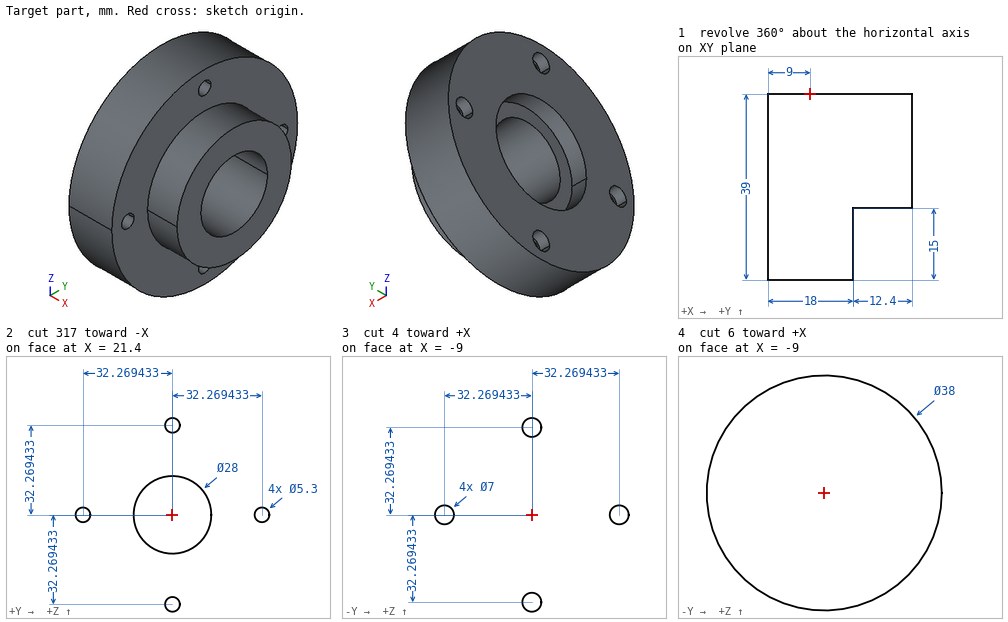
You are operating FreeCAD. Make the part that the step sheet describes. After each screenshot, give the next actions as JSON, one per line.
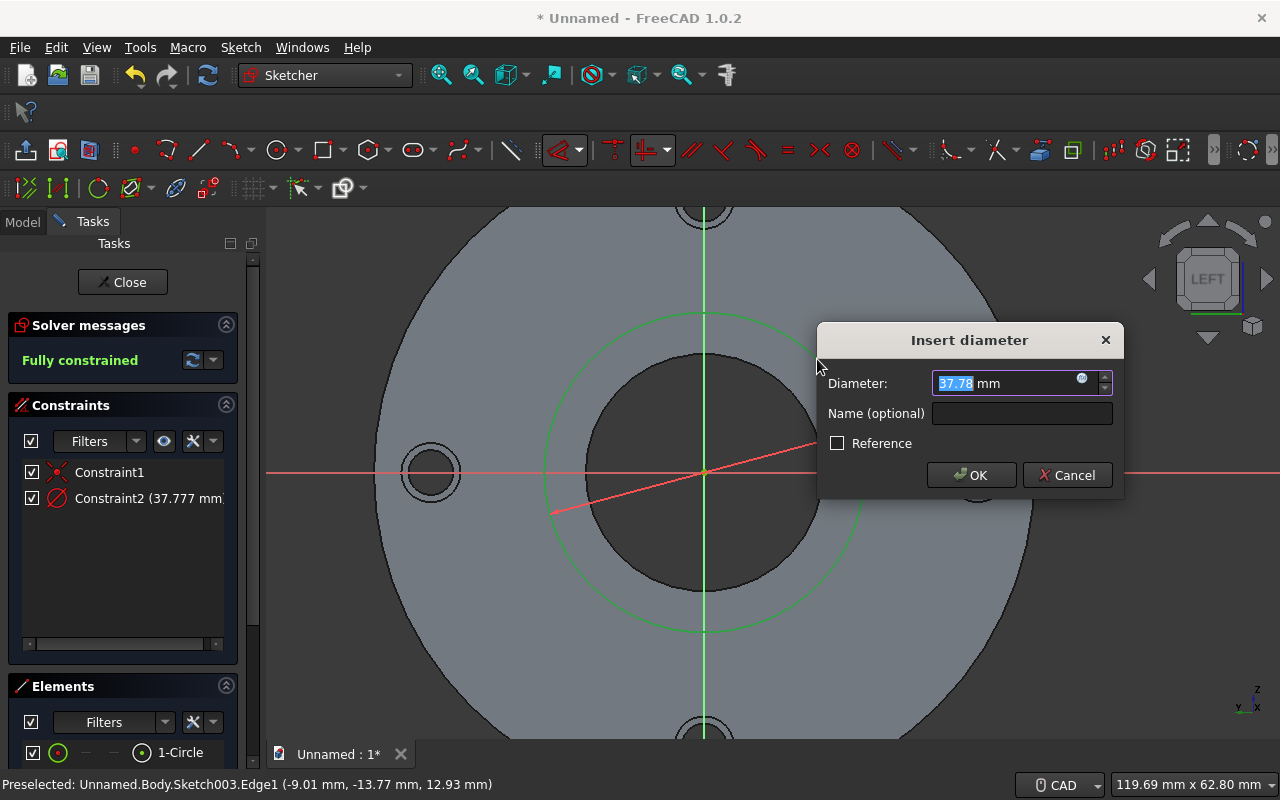
{"action": "type", "text": "38"}
{"action": "key", "text": "Return"}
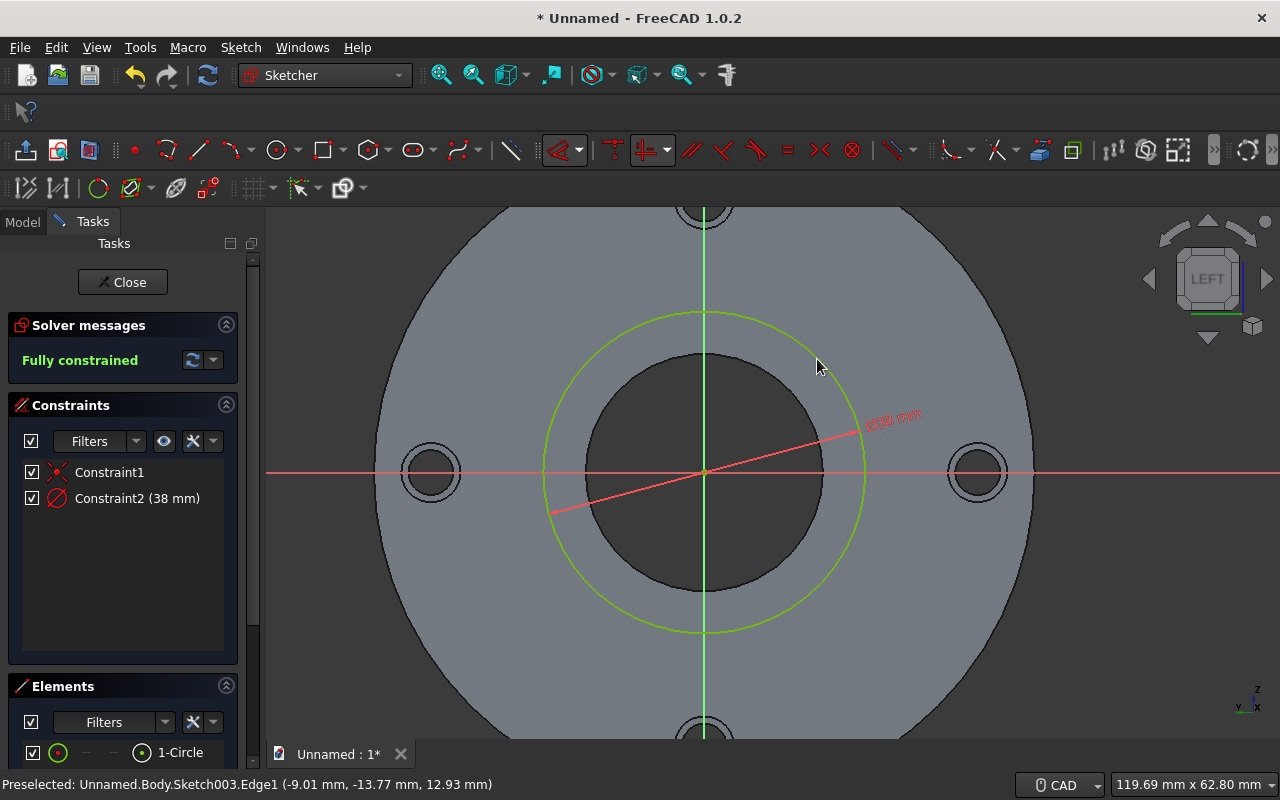
{"action": "left_click", "coordinate": [123, 282]}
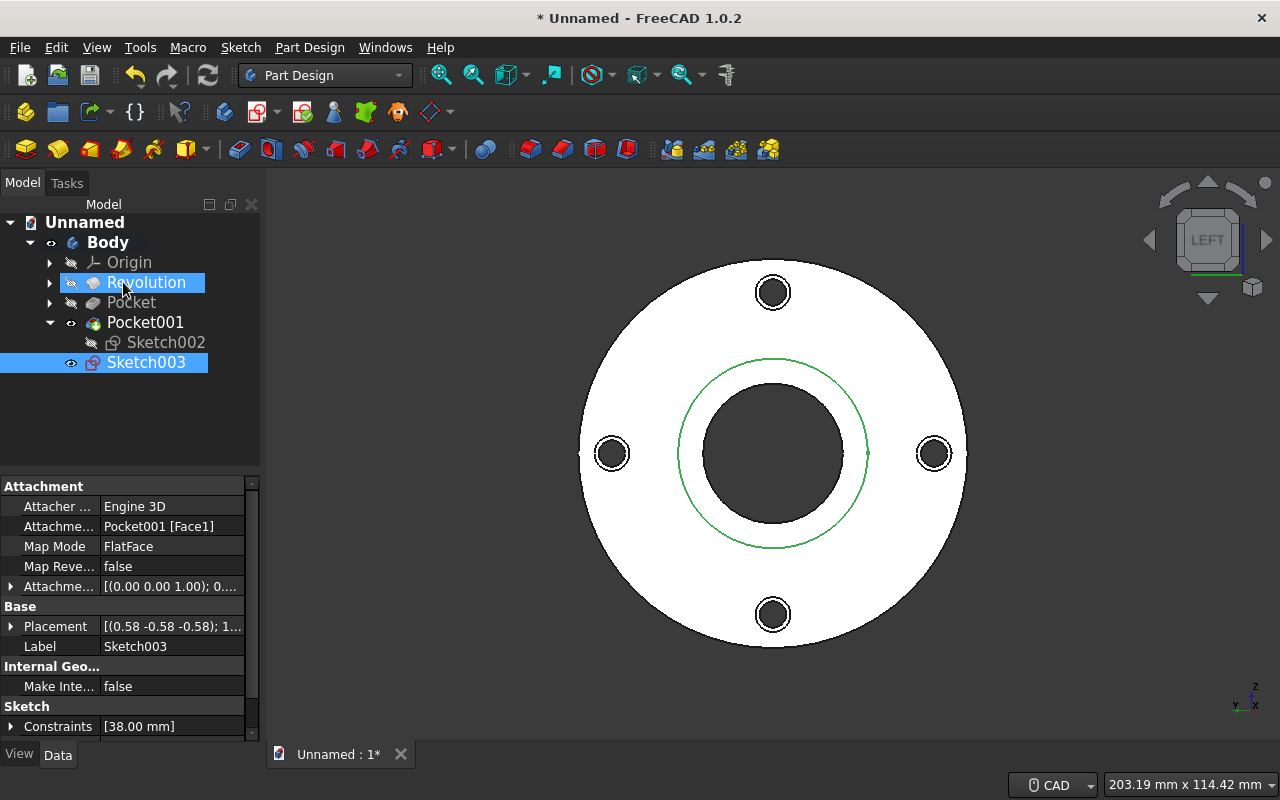
{"action": "left_click", "coordinate": [240, 150]}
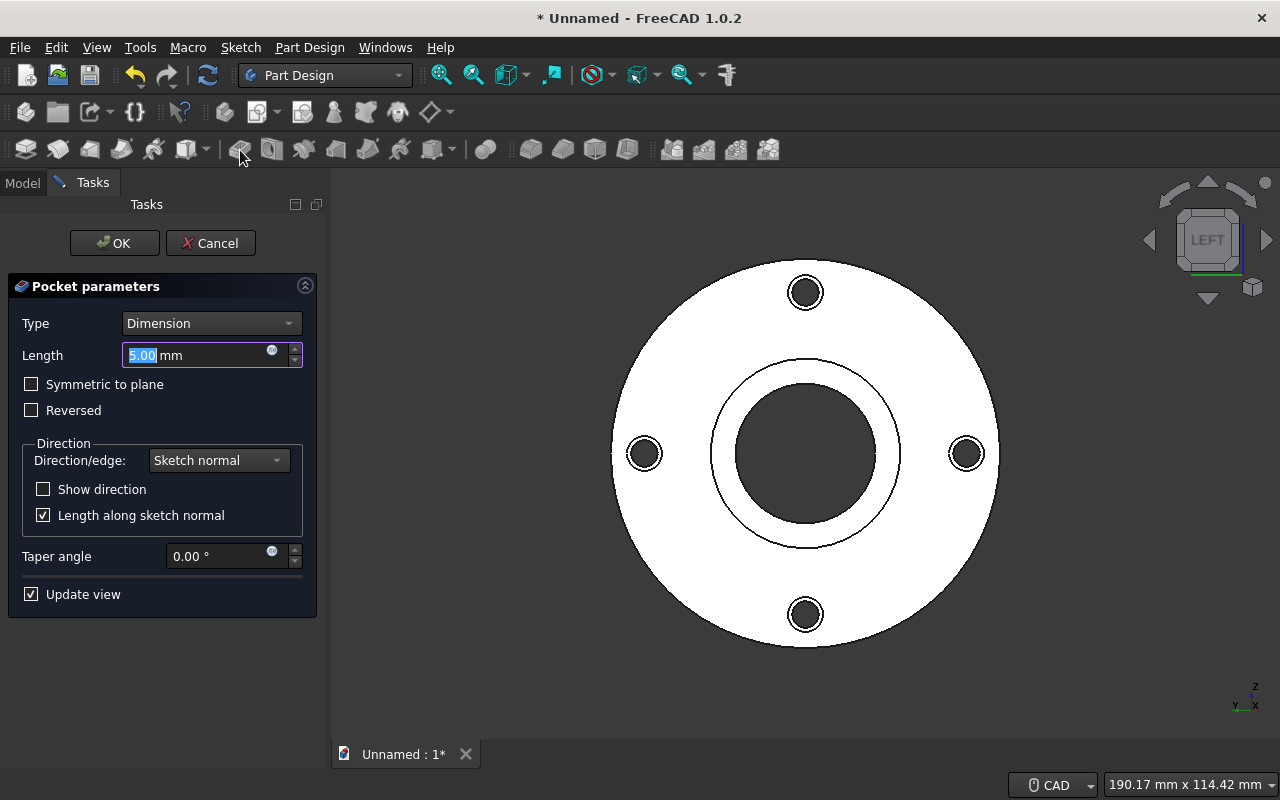
{"action": "type", "text": "6"}
{"action": "key", "text": "Tab"}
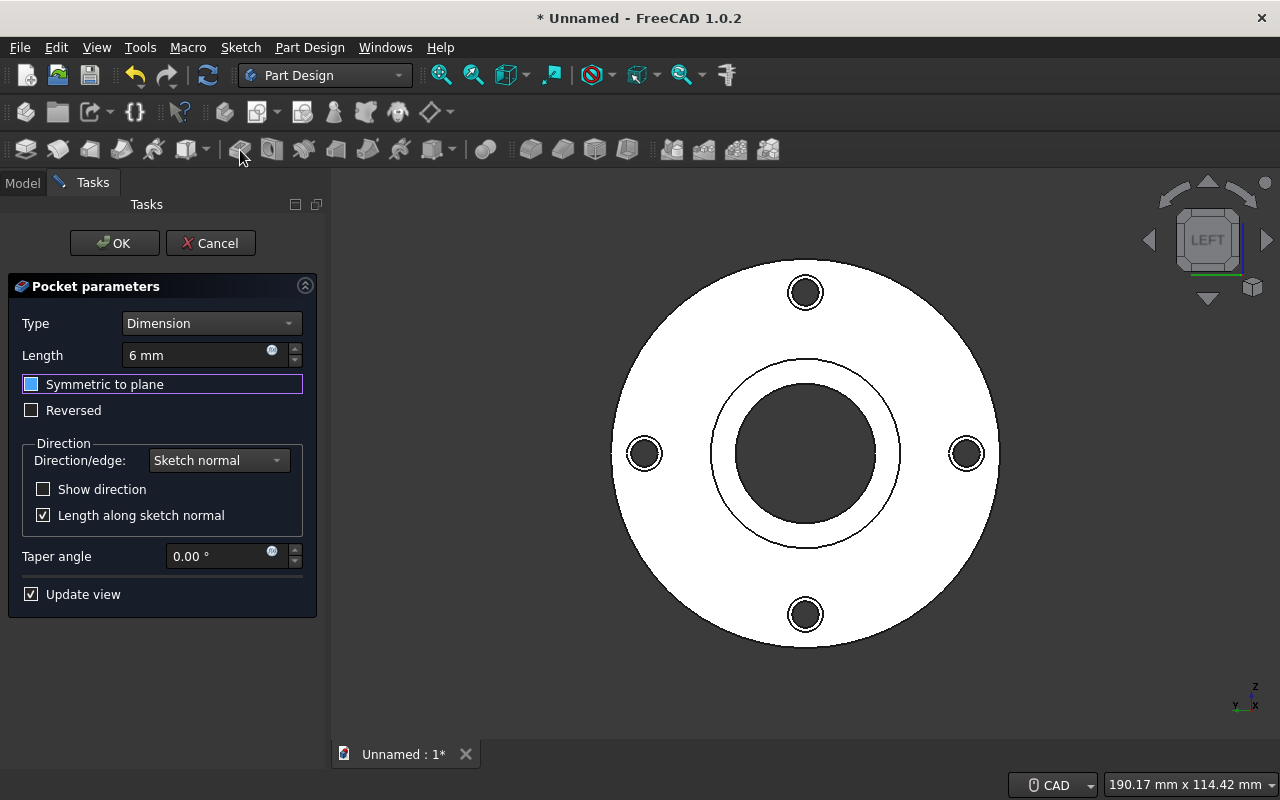
{"action": "left_click", "coordinate": [115, 243]}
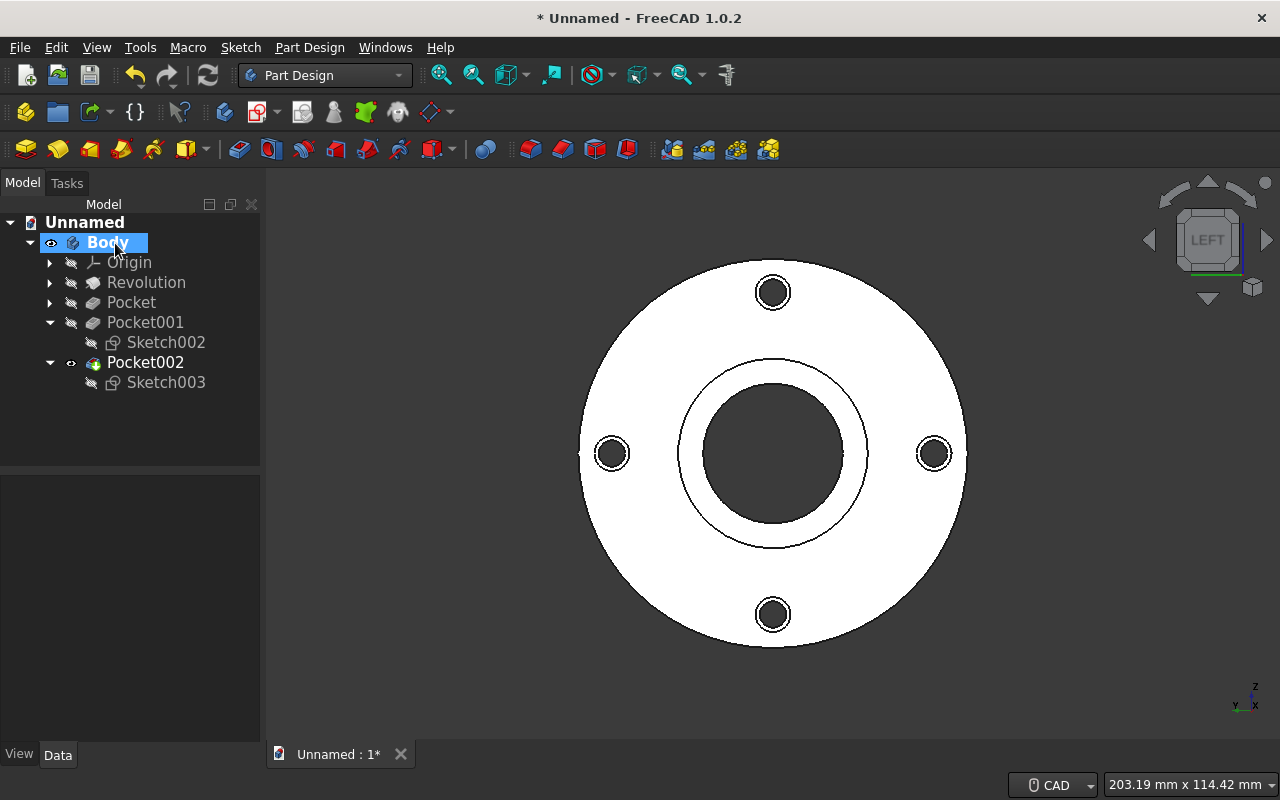
{"action": "key", "text": "0"}